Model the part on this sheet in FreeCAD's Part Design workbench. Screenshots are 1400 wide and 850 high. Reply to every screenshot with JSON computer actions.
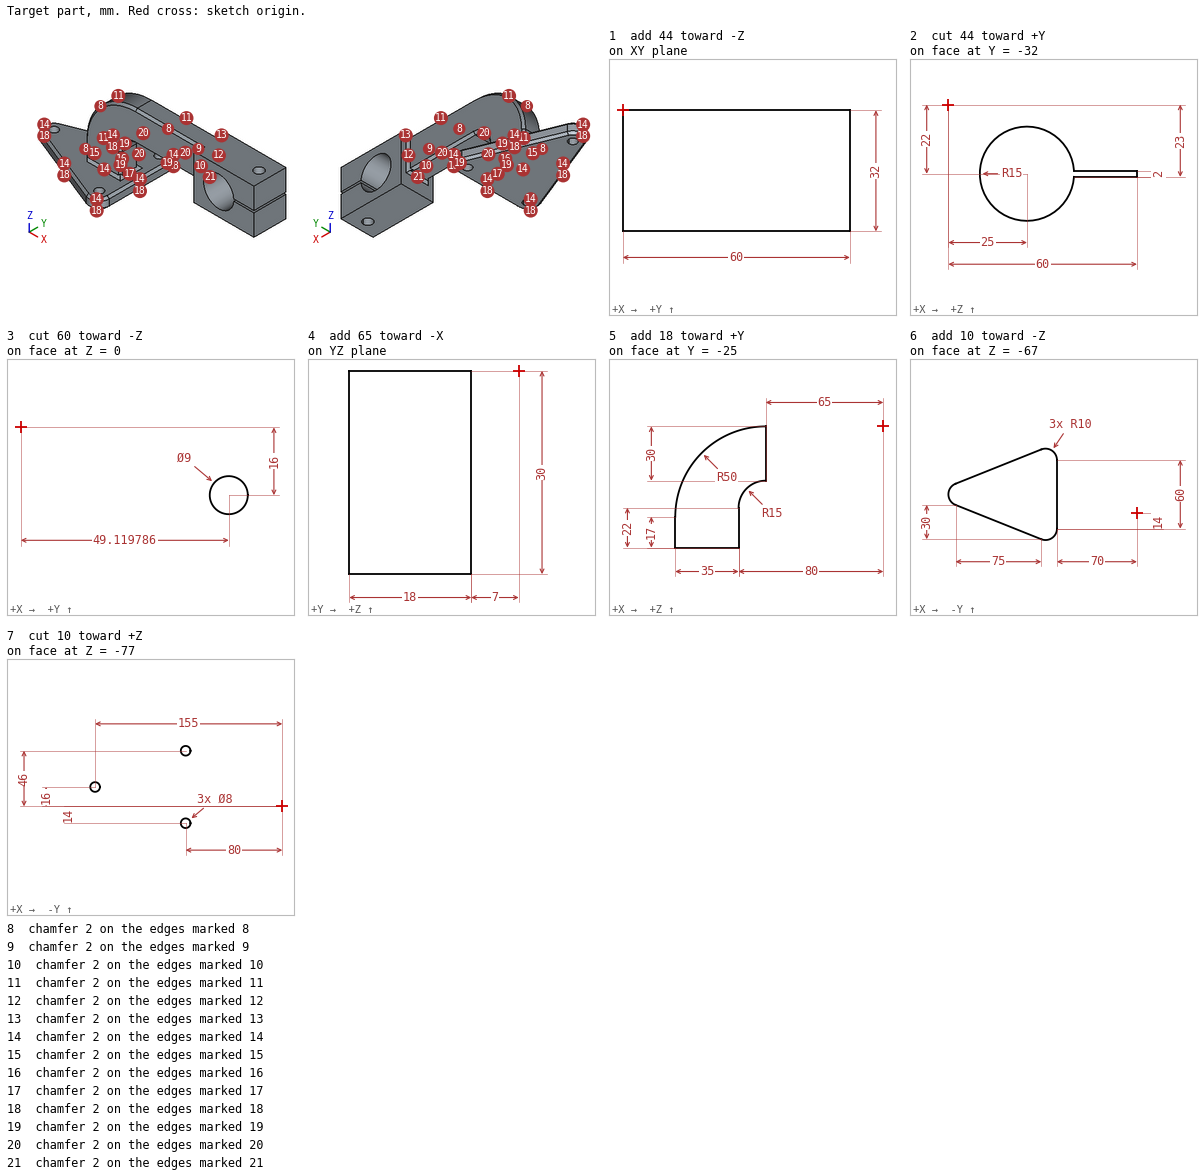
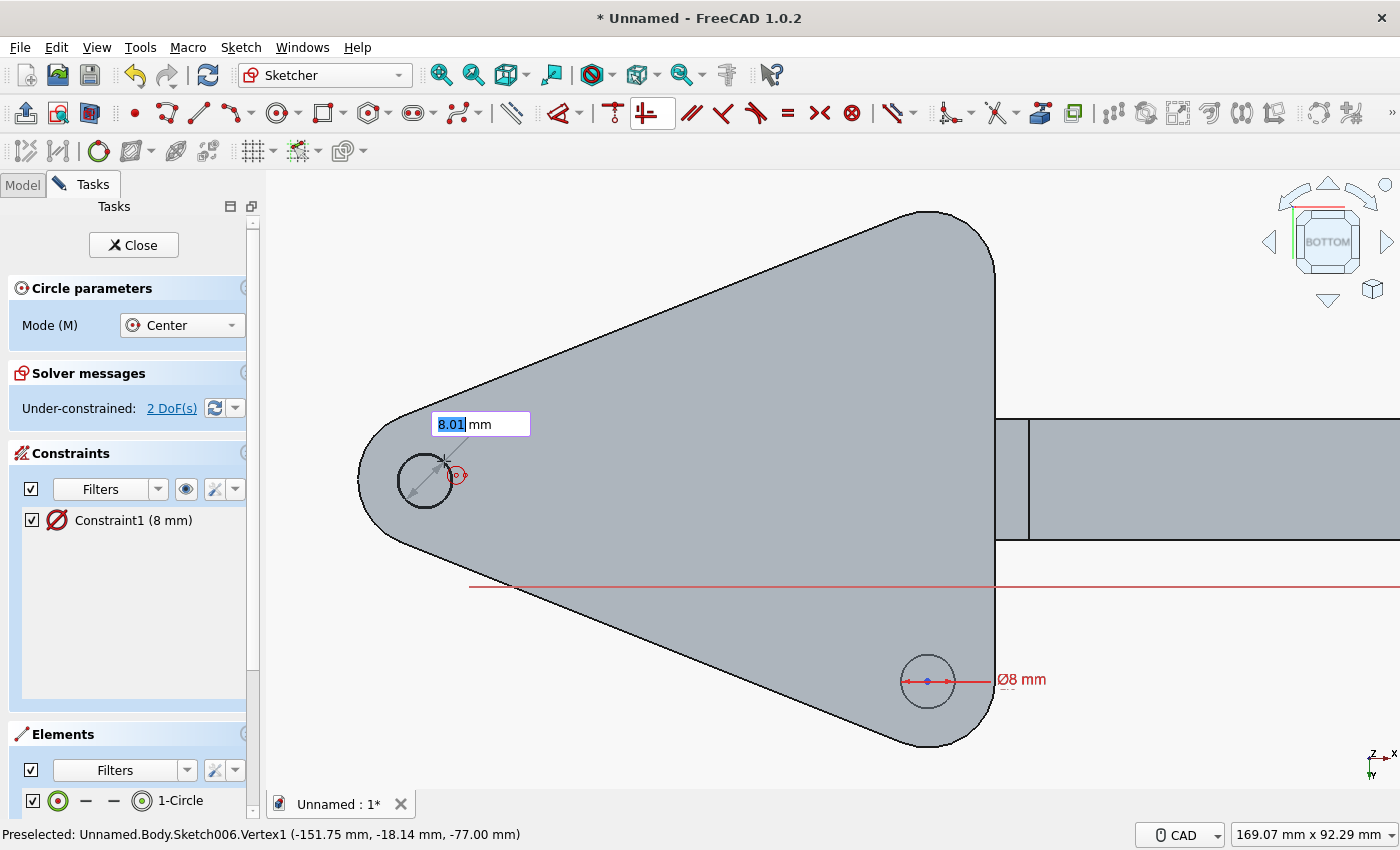
{"action": "type", "text": "8"}
{"action": "key", "text": "Return"}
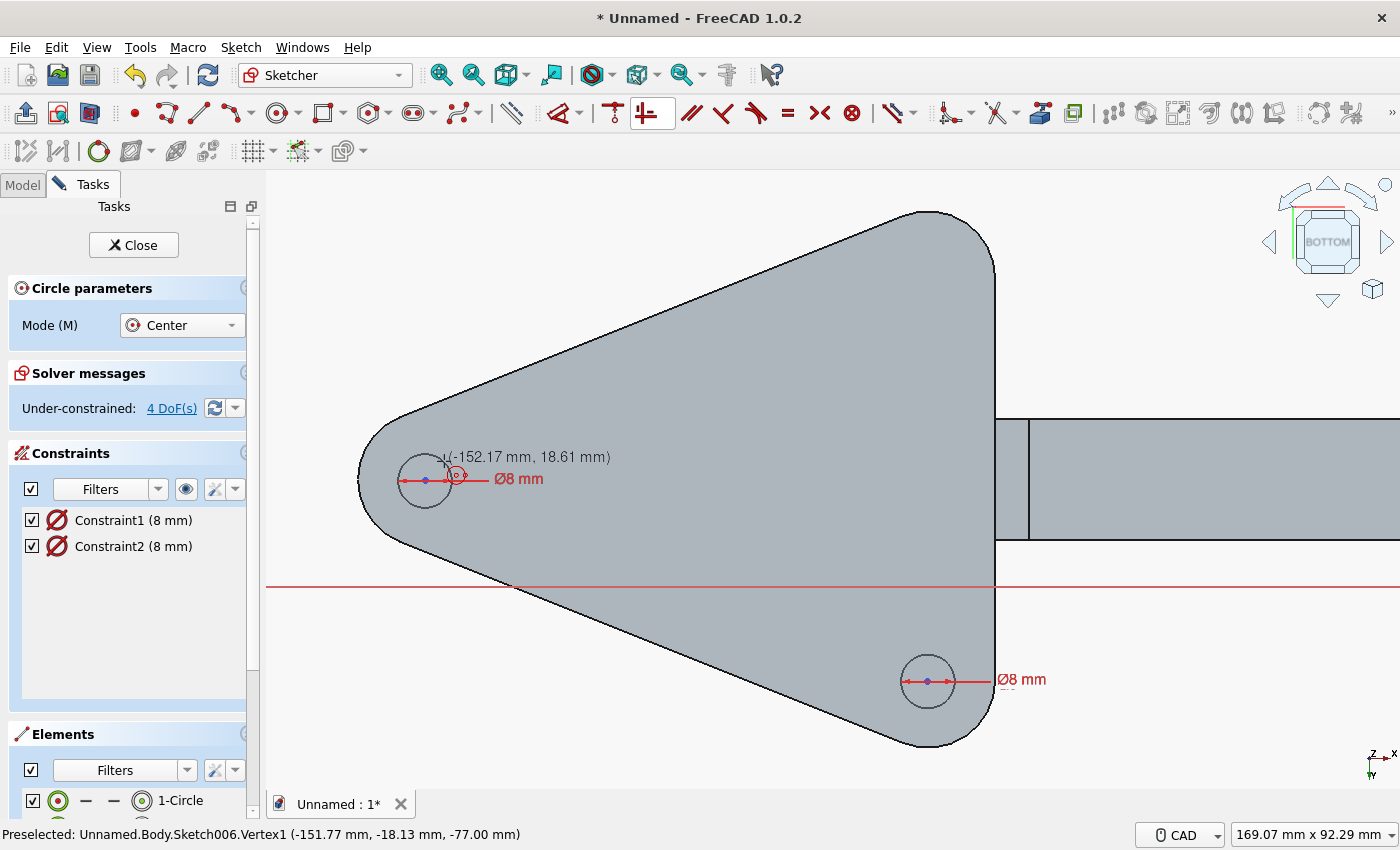
{"action": "left_click", "coordinate": [928, 278]}
{"action": "mouse_move", "coordinate": [947, 259]}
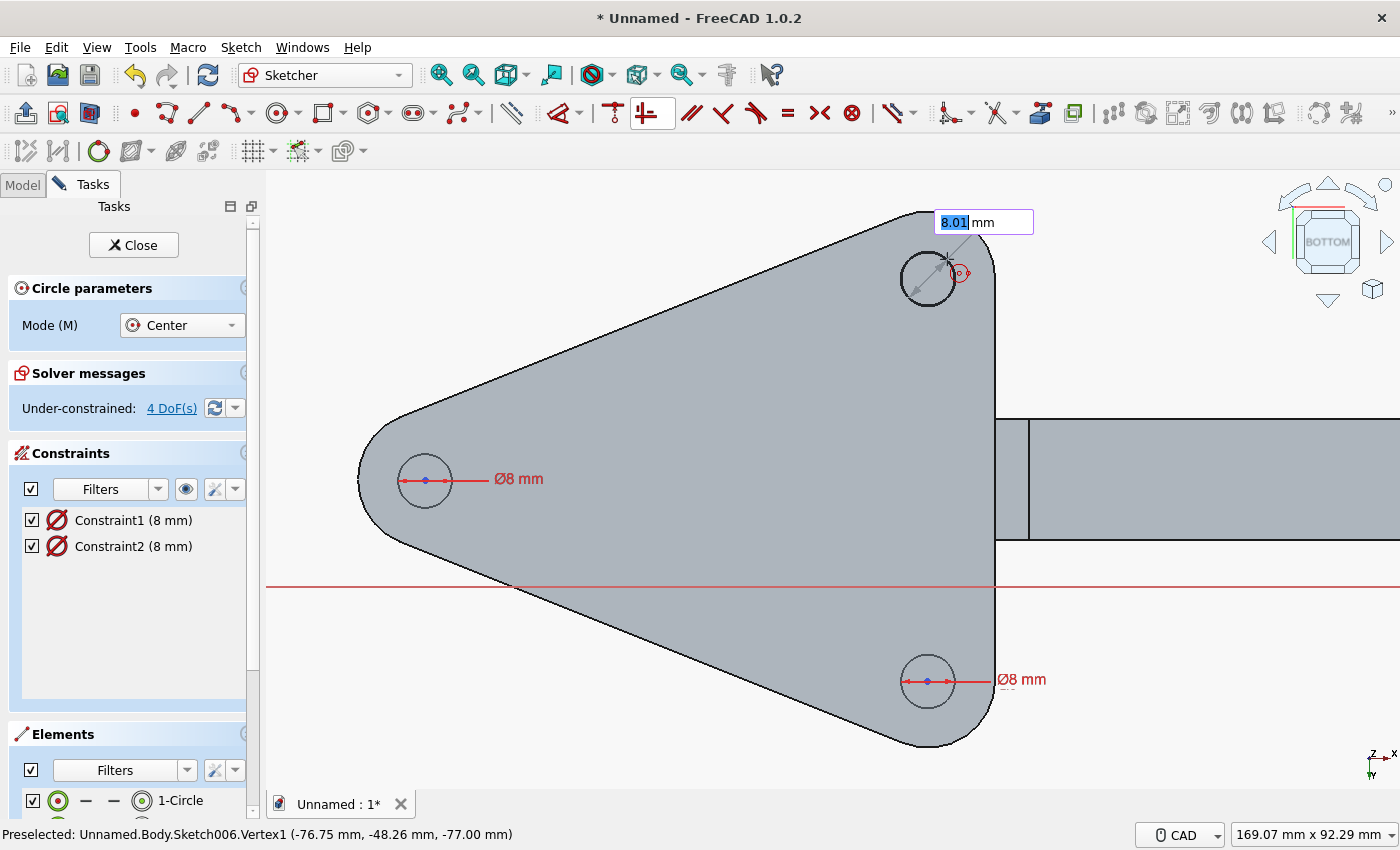
{"action": "type", "text": "8"}
{"action": "key", "text": "Return"}
{"action": "key", "text": "Escape"}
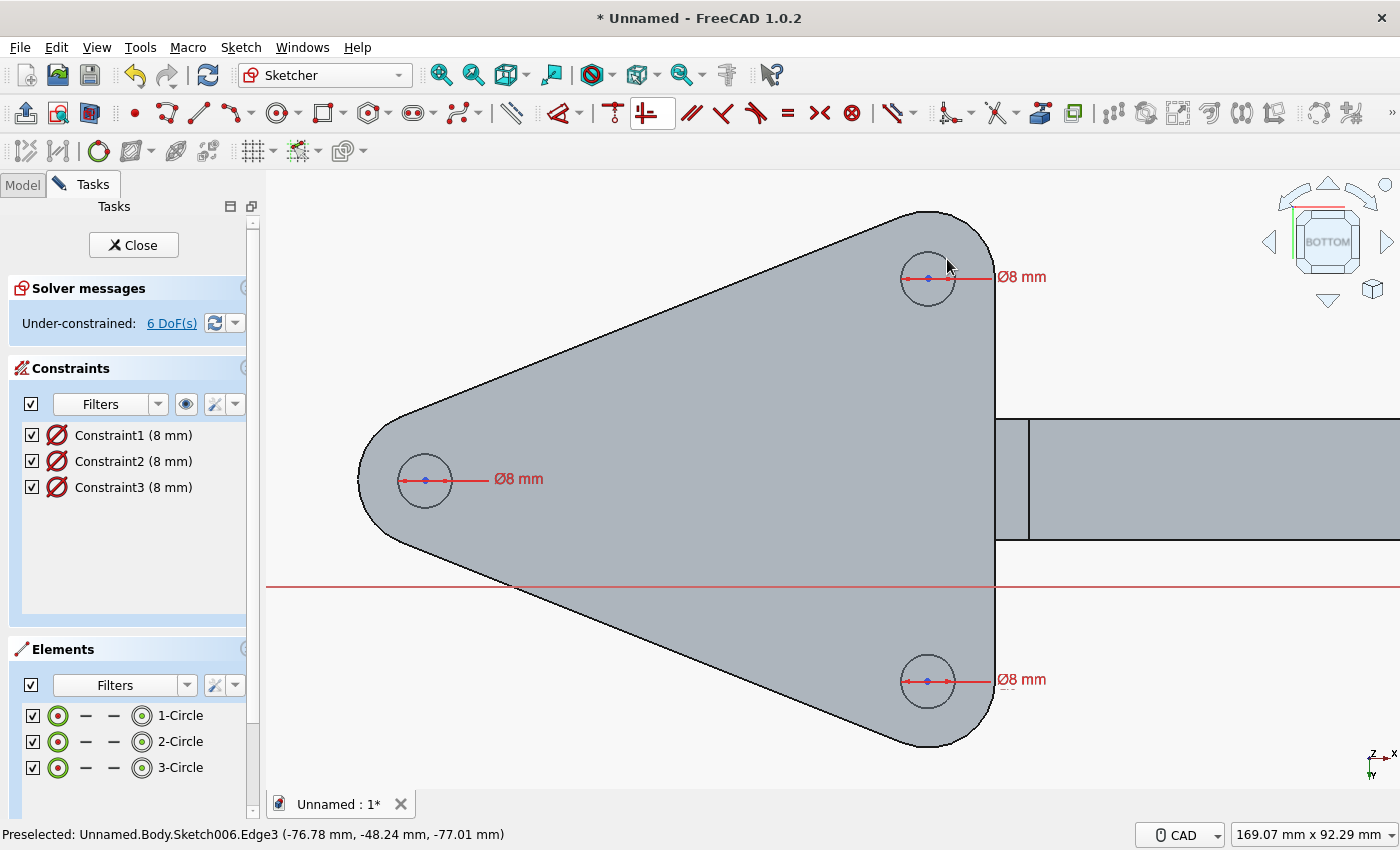
{"action": "left_click", "coordinate": [928, 682]}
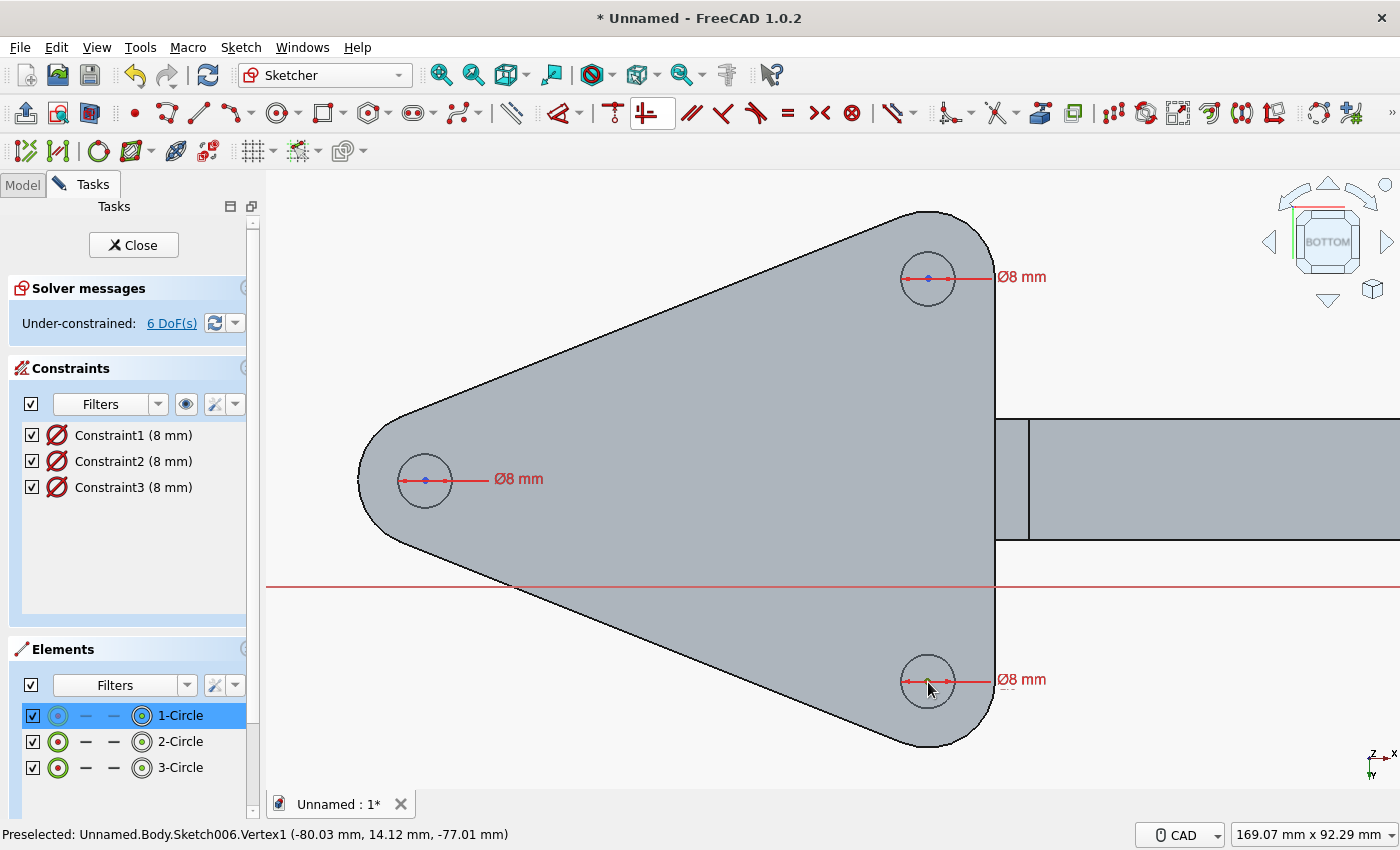
{"action": "left_click", "coordinate": [928, 279]}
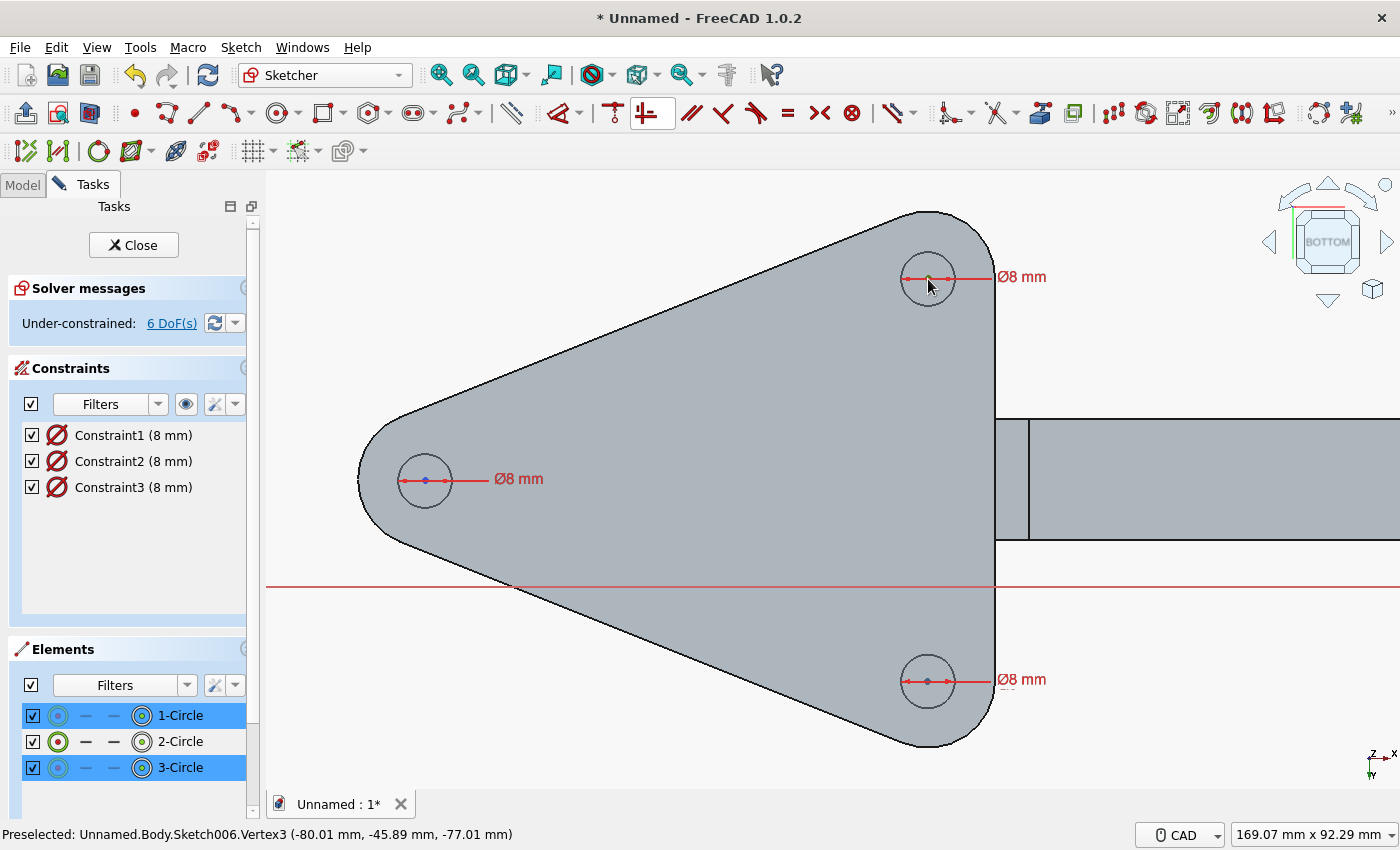
{"action": "left_click", "coordinate": [670, 114]}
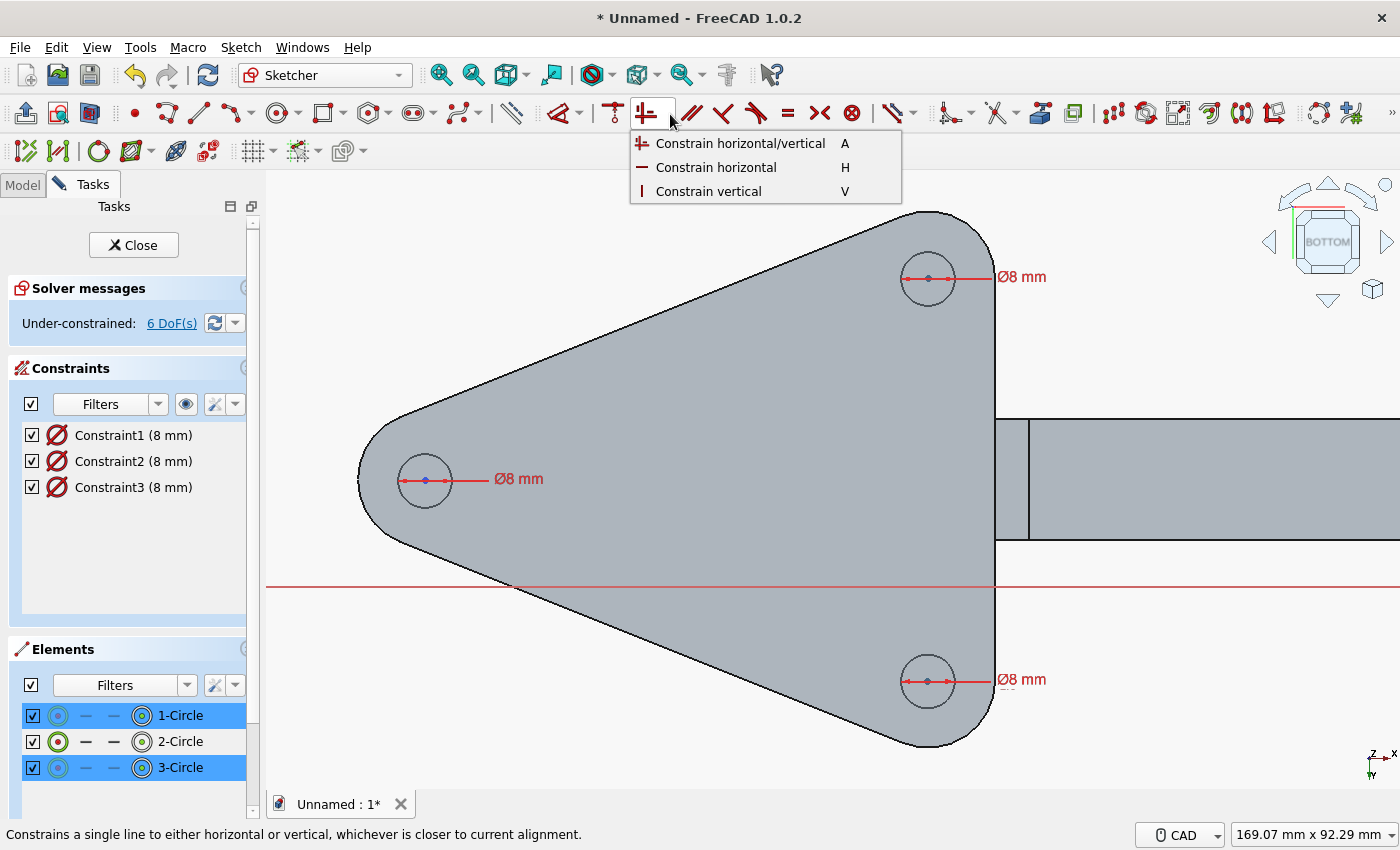
{"action": "left_click", "coordinate": [766, 191]}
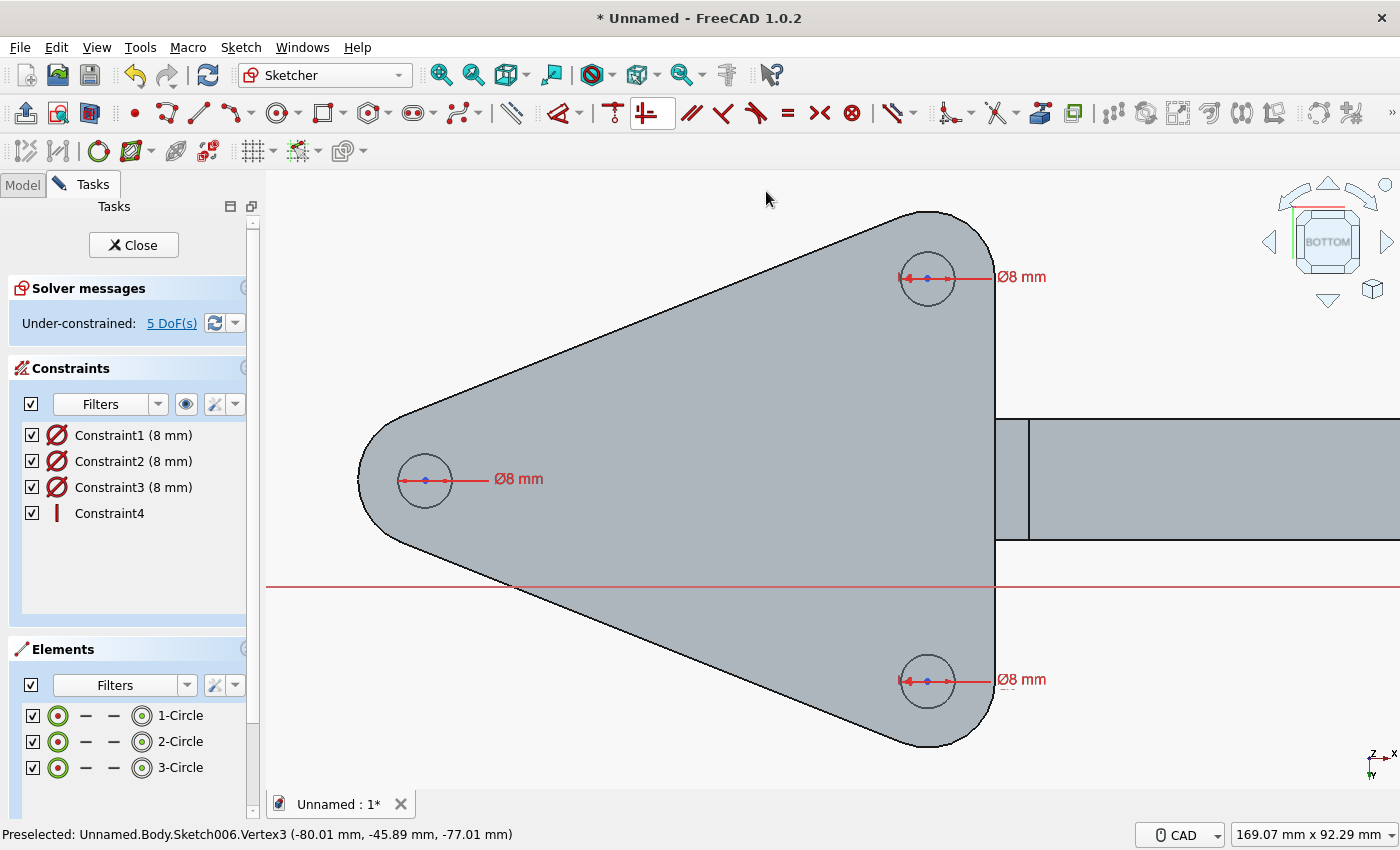
{"action": "left_click", "coordinate": [558, 114]}